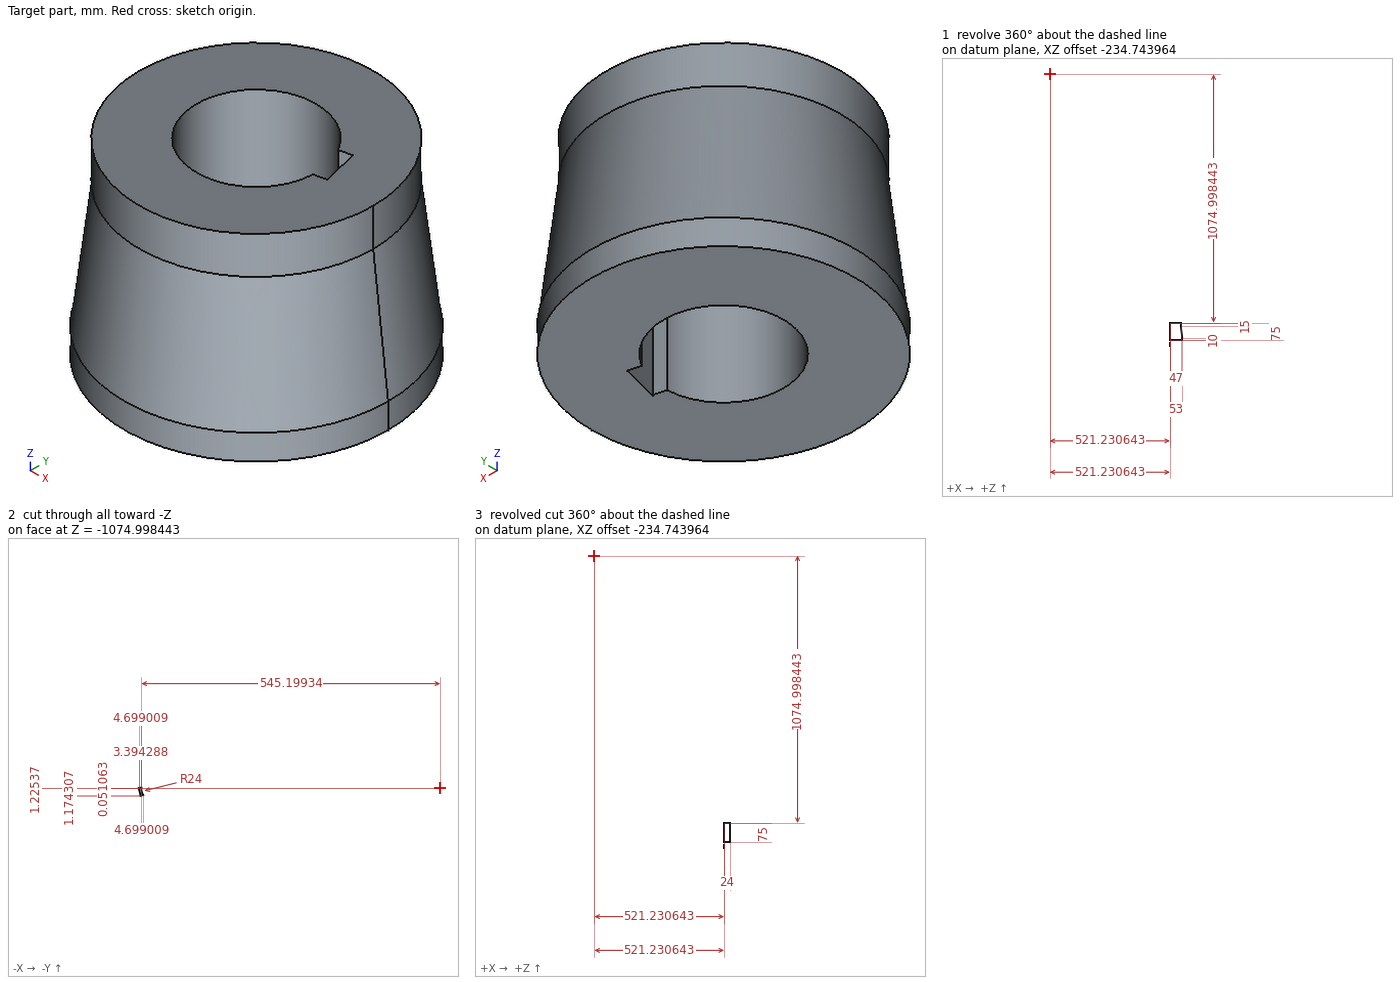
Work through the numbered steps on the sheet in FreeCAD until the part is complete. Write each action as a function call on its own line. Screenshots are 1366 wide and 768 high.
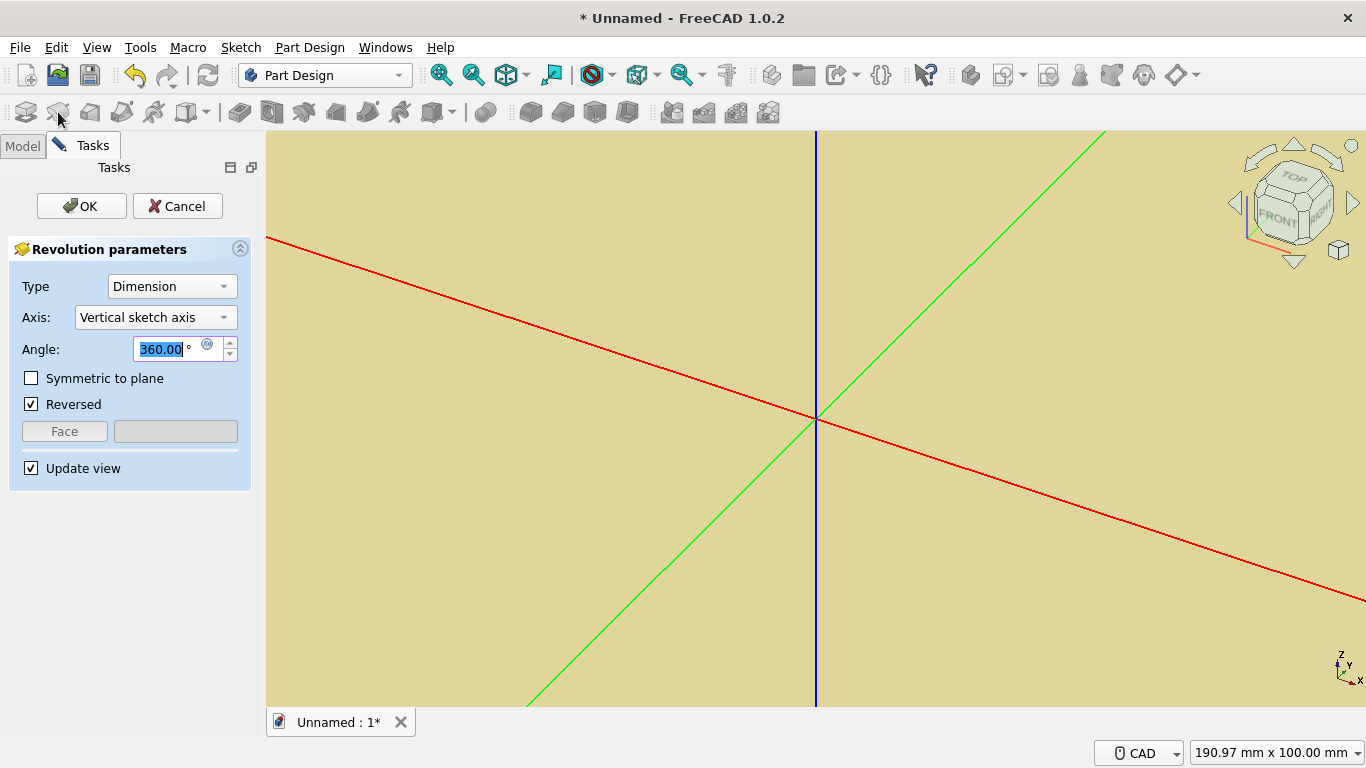
click(156, 318)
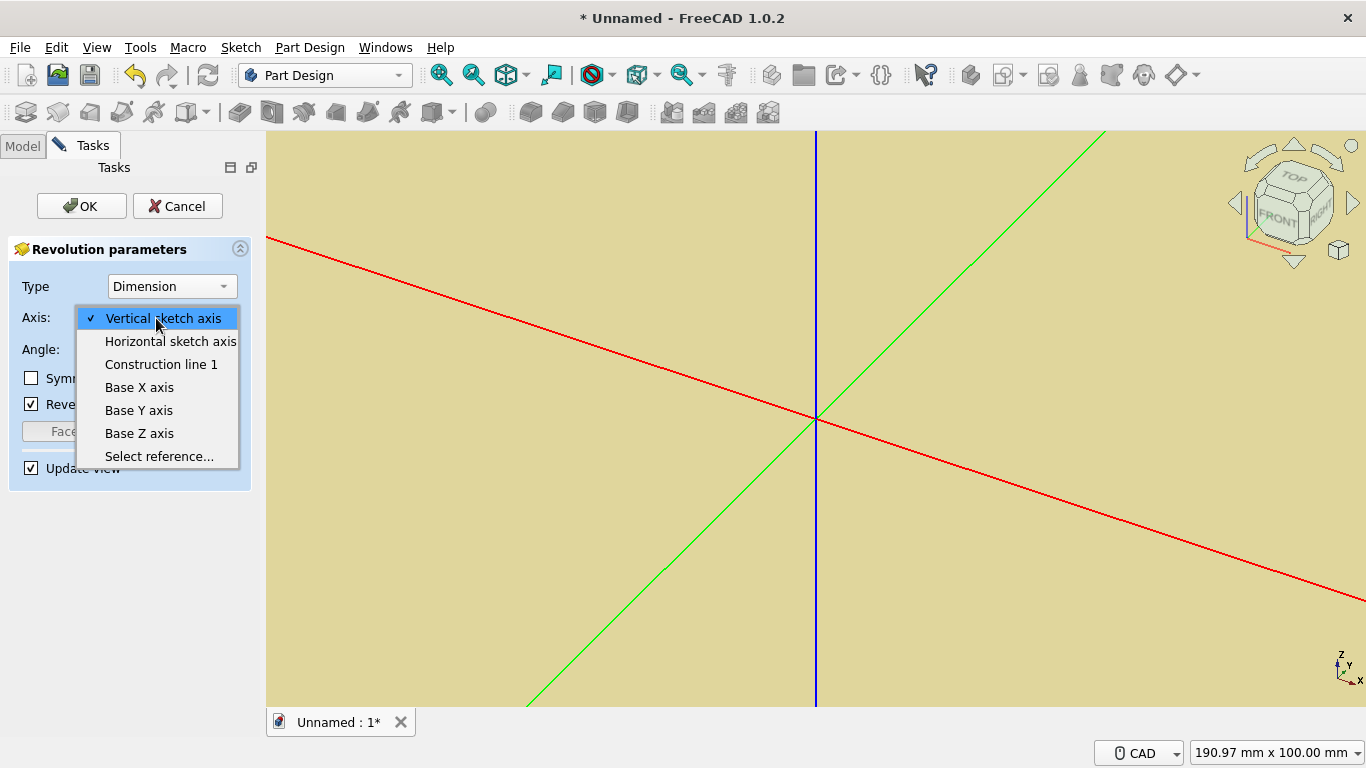
click(156, 364)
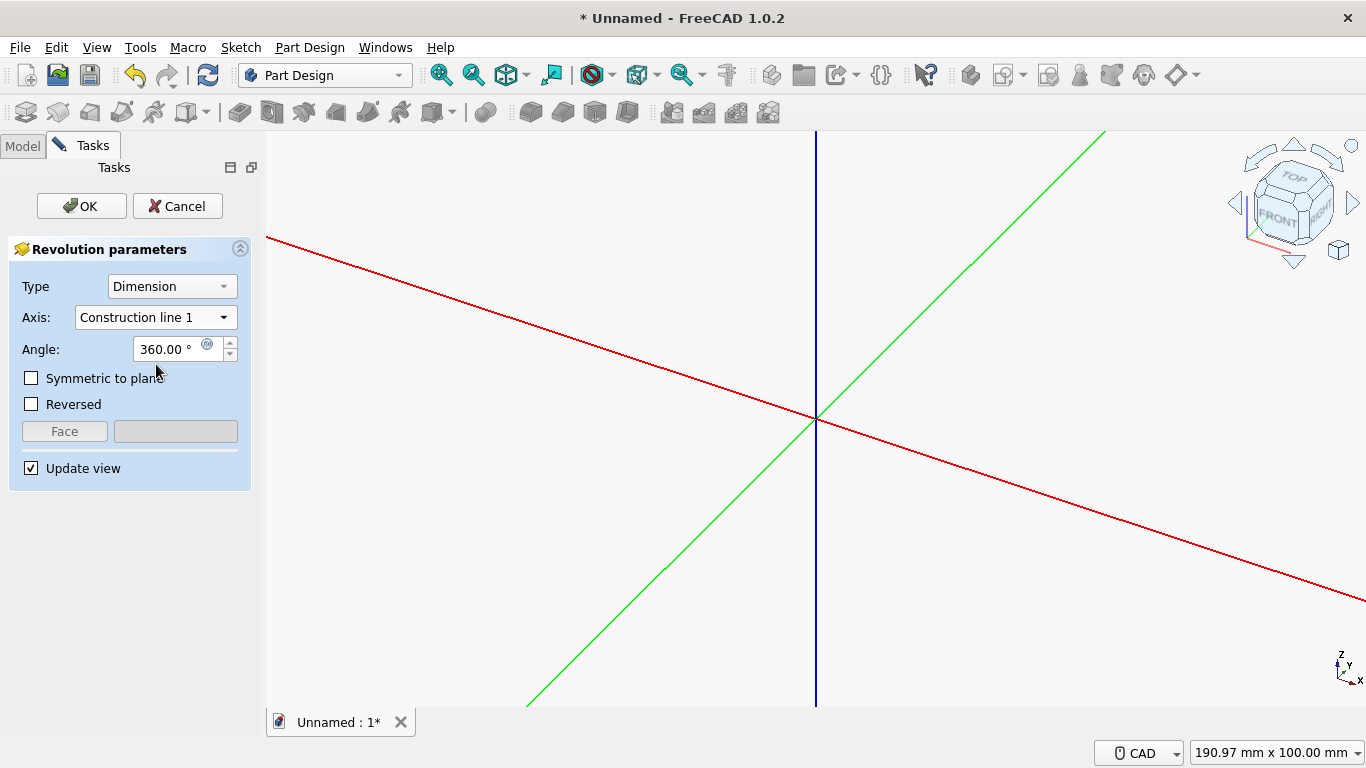
click(82, 206)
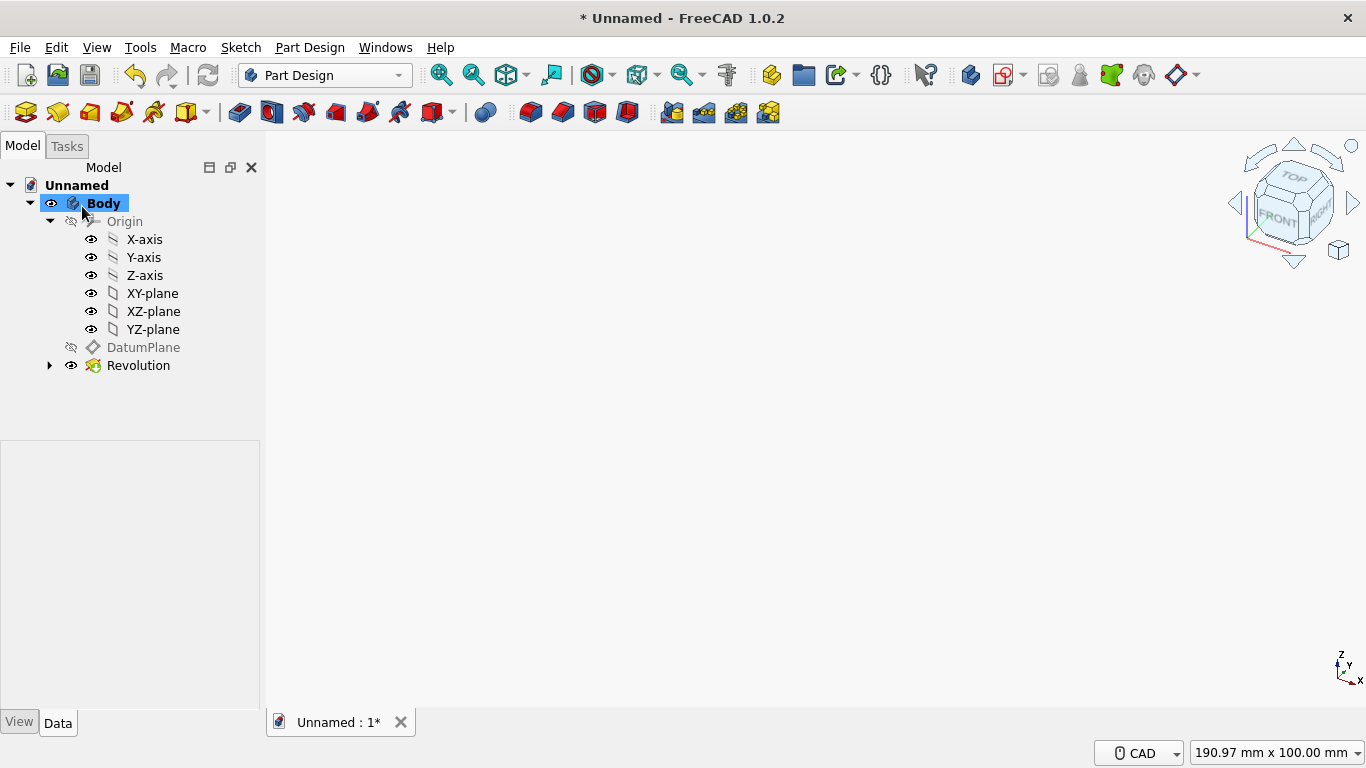
click(442, 76)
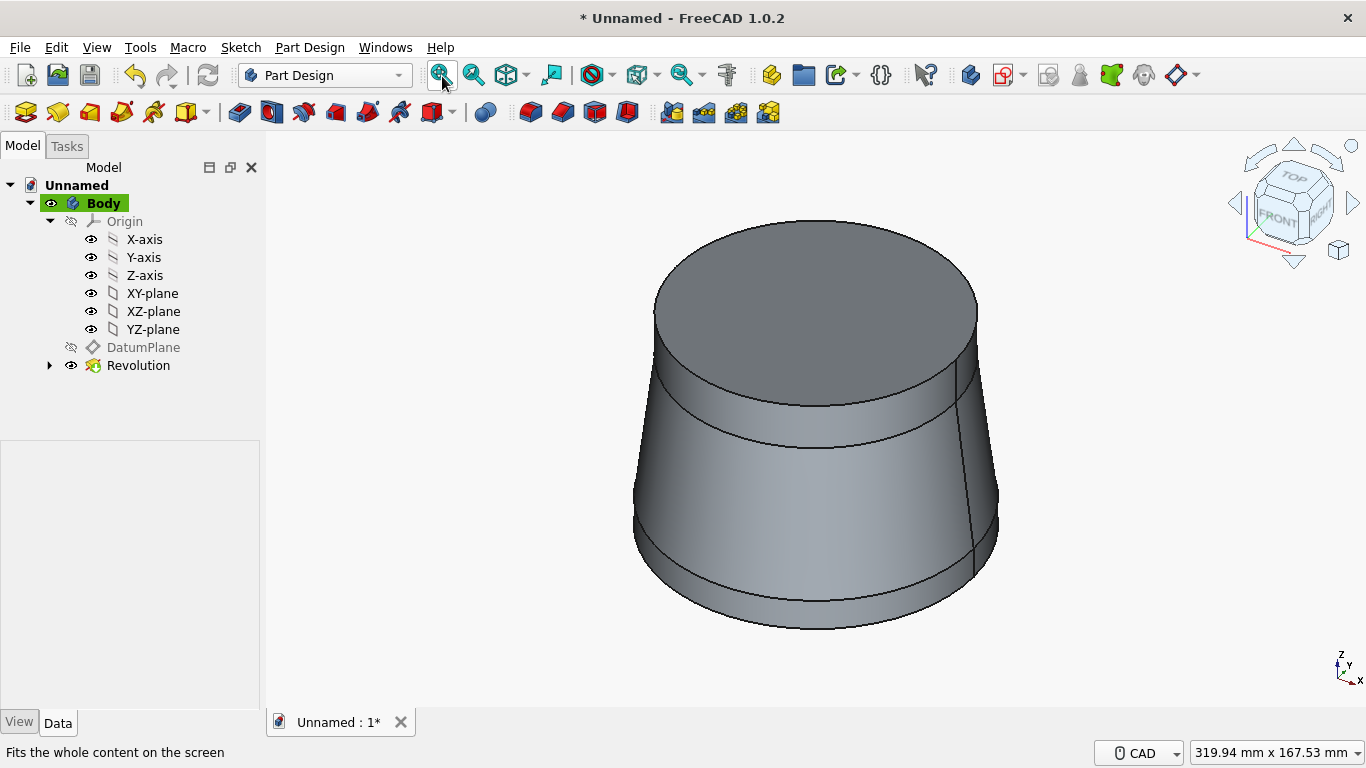
click(816, 312)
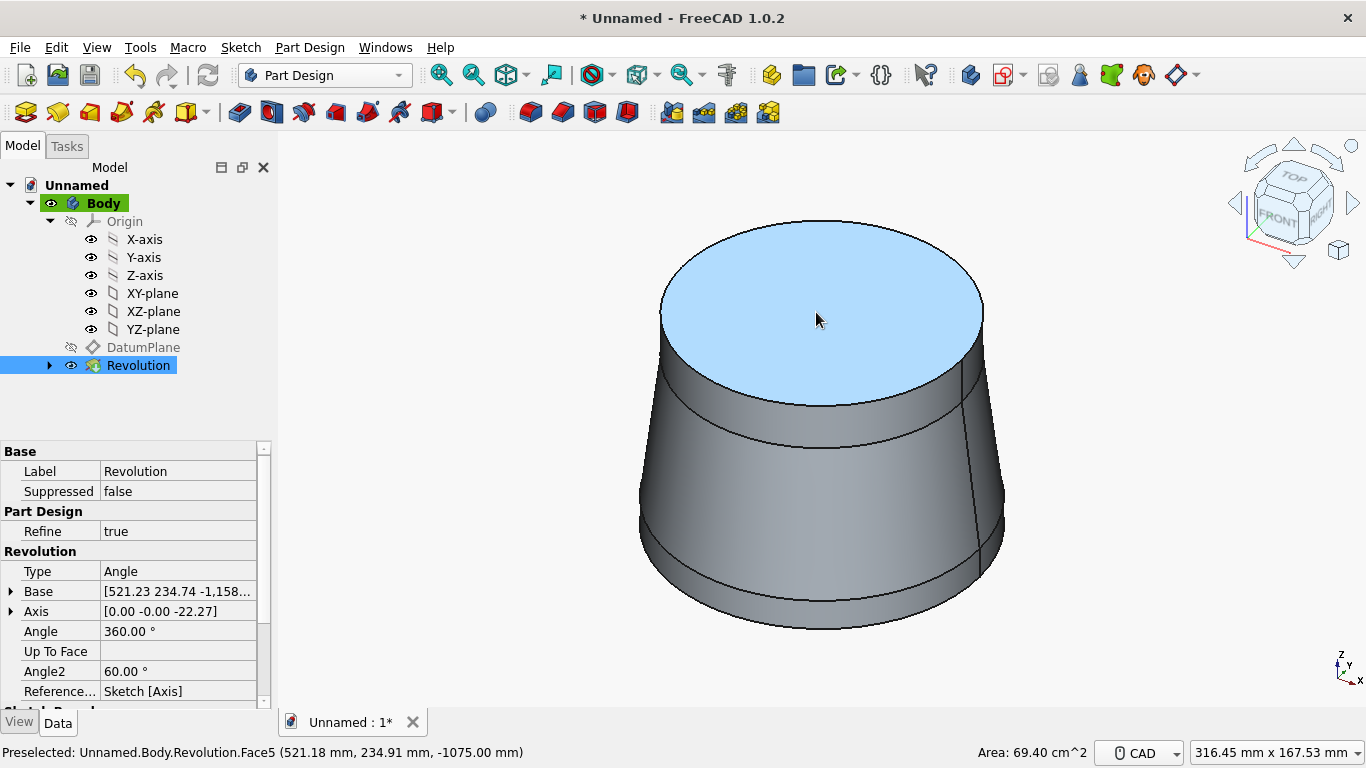
click(1004, 76)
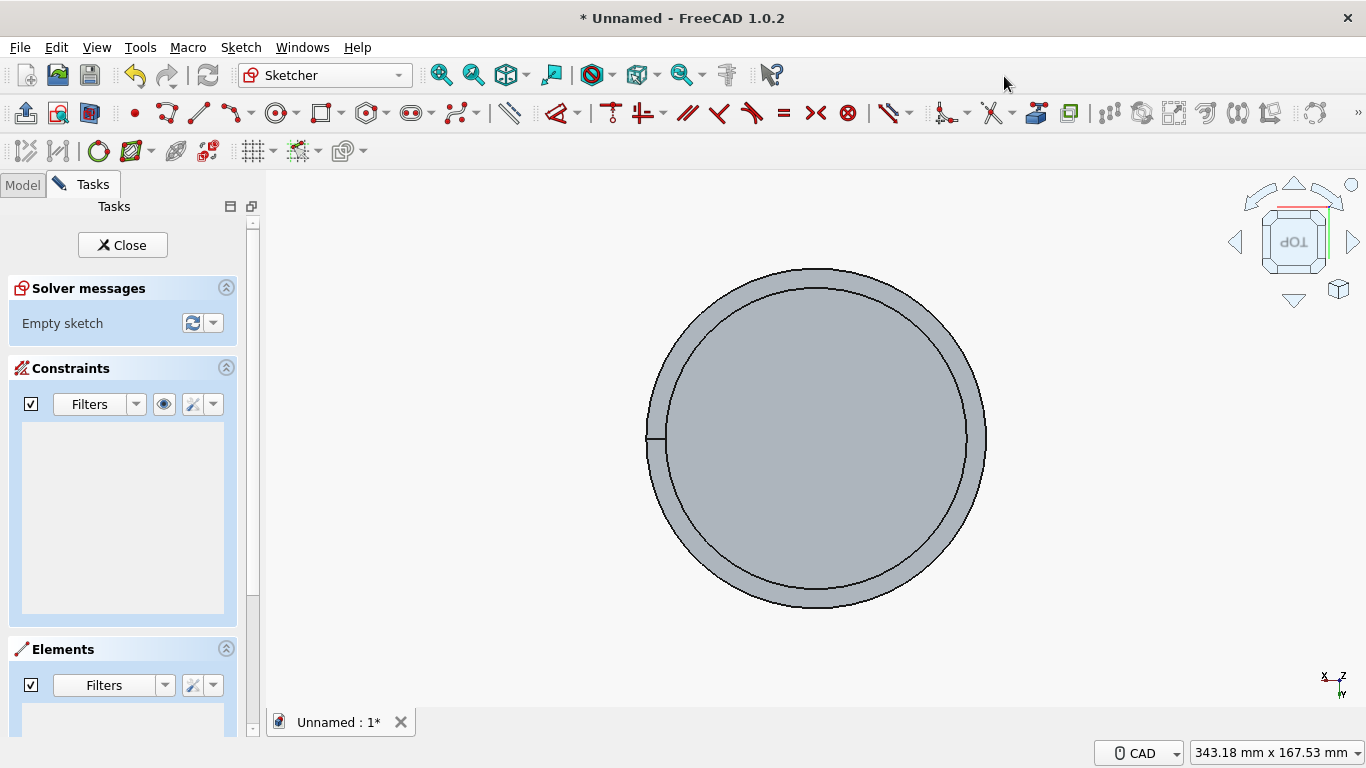
scroll(736, 461, up, 10)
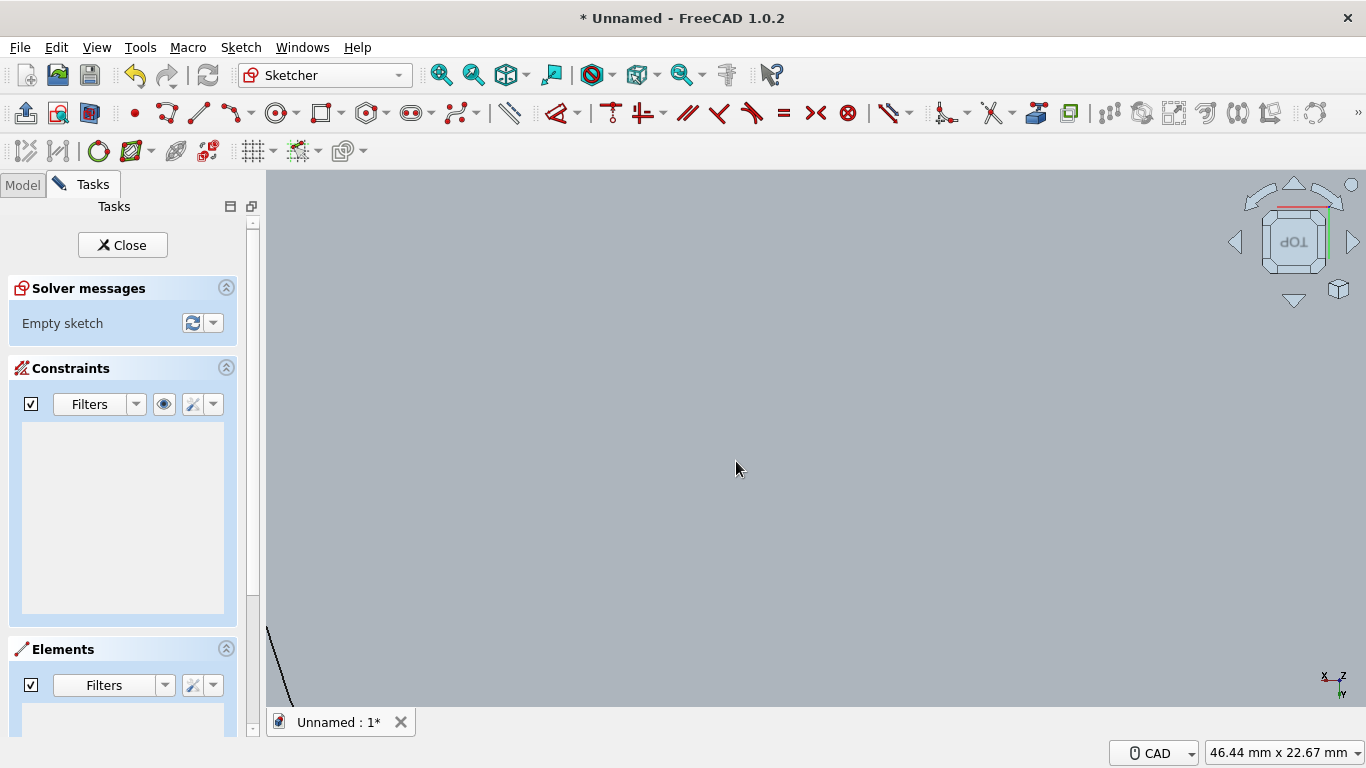
click(168, 114)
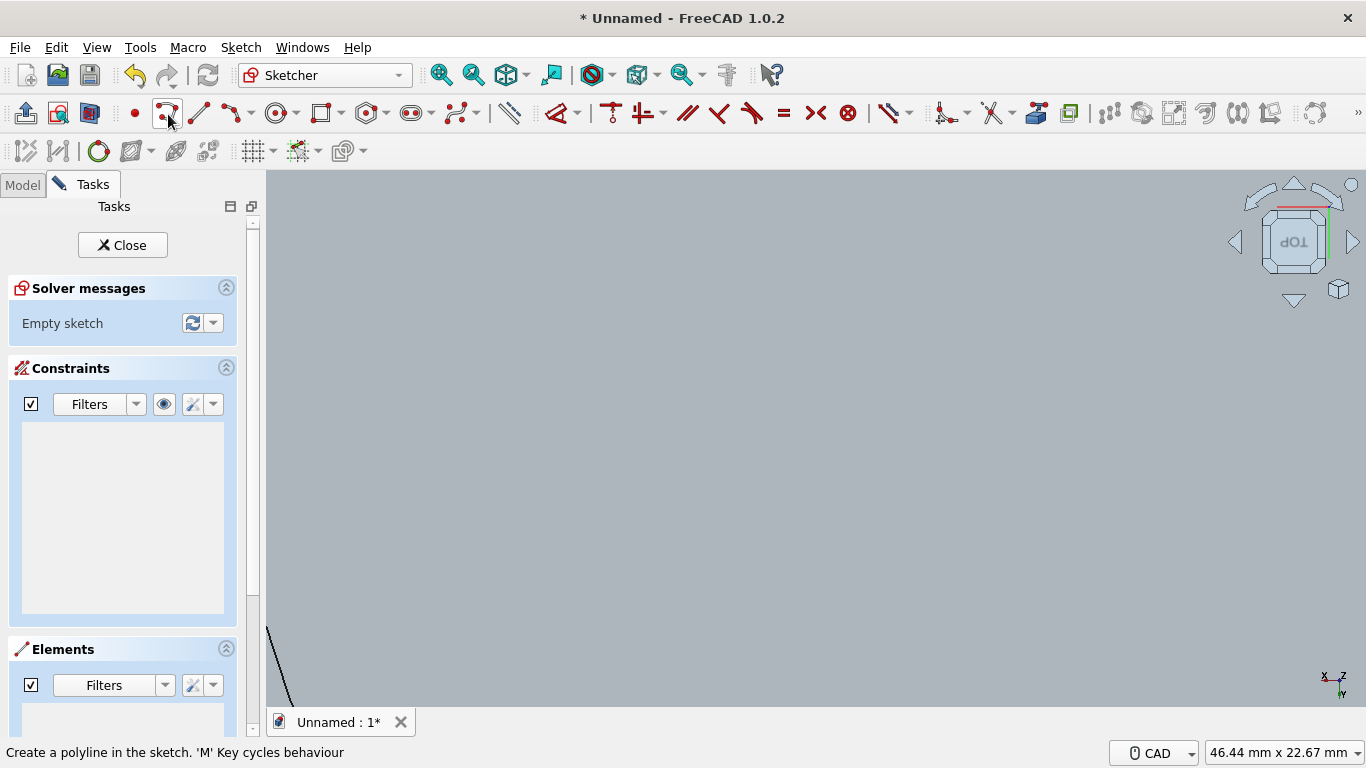
click(758, 262)